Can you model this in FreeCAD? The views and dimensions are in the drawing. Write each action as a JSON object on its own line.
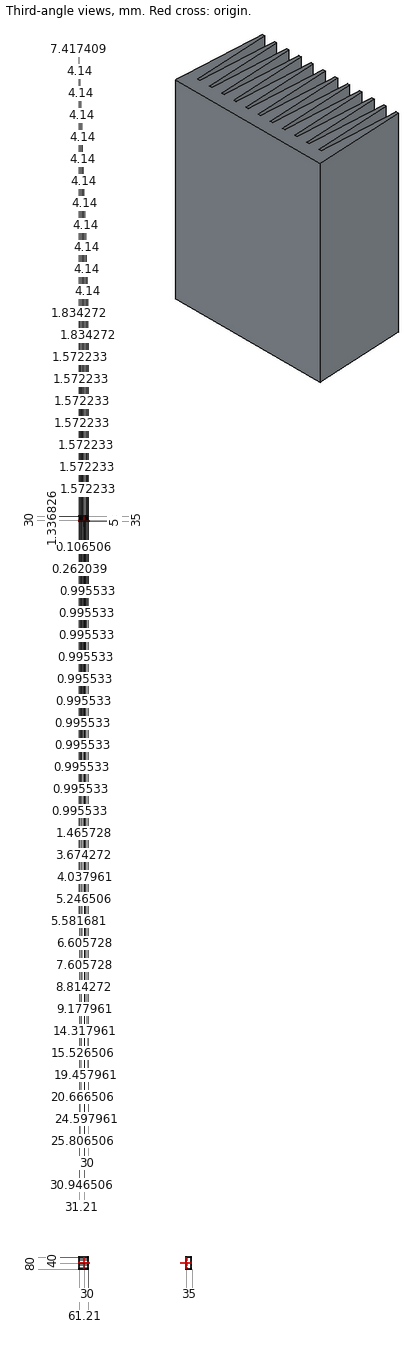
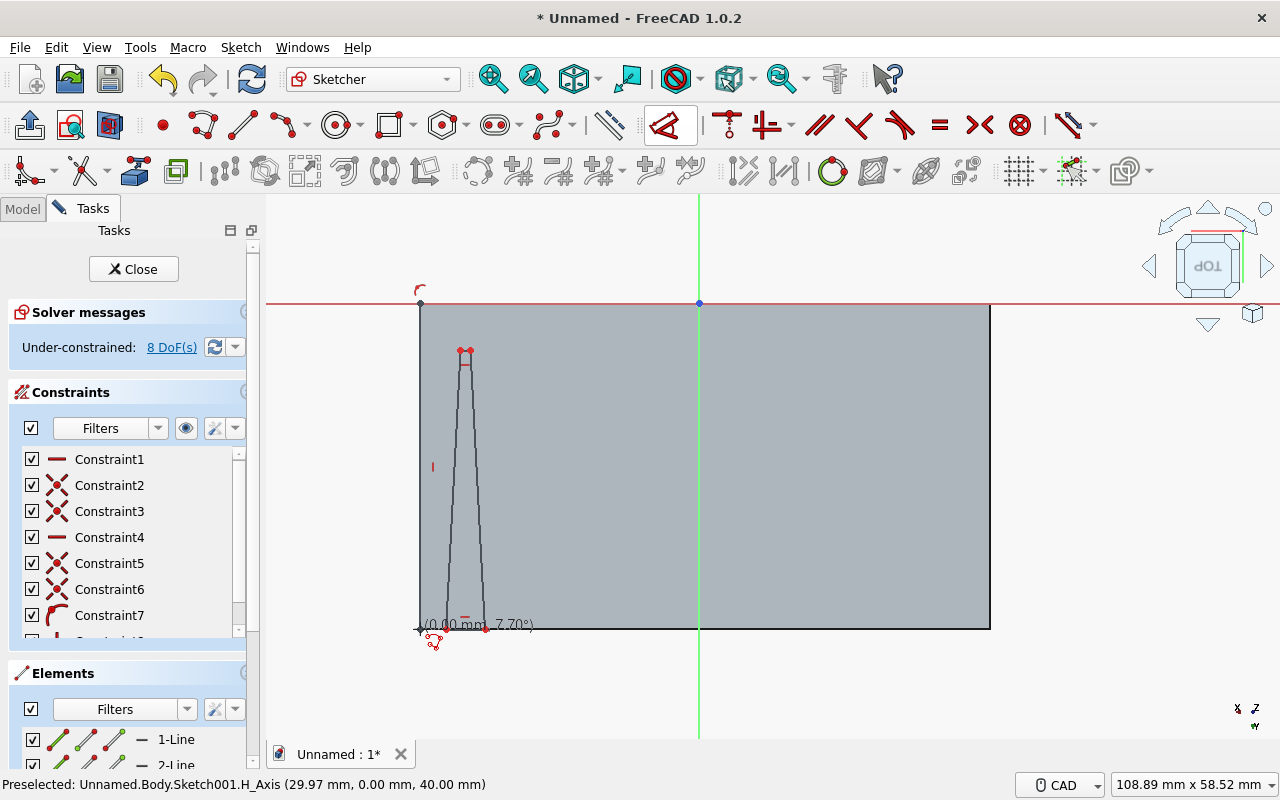
{"action": "scroll", "coordinate": [437, 629], "scroll_direction": "up", "scroll_amount": 3}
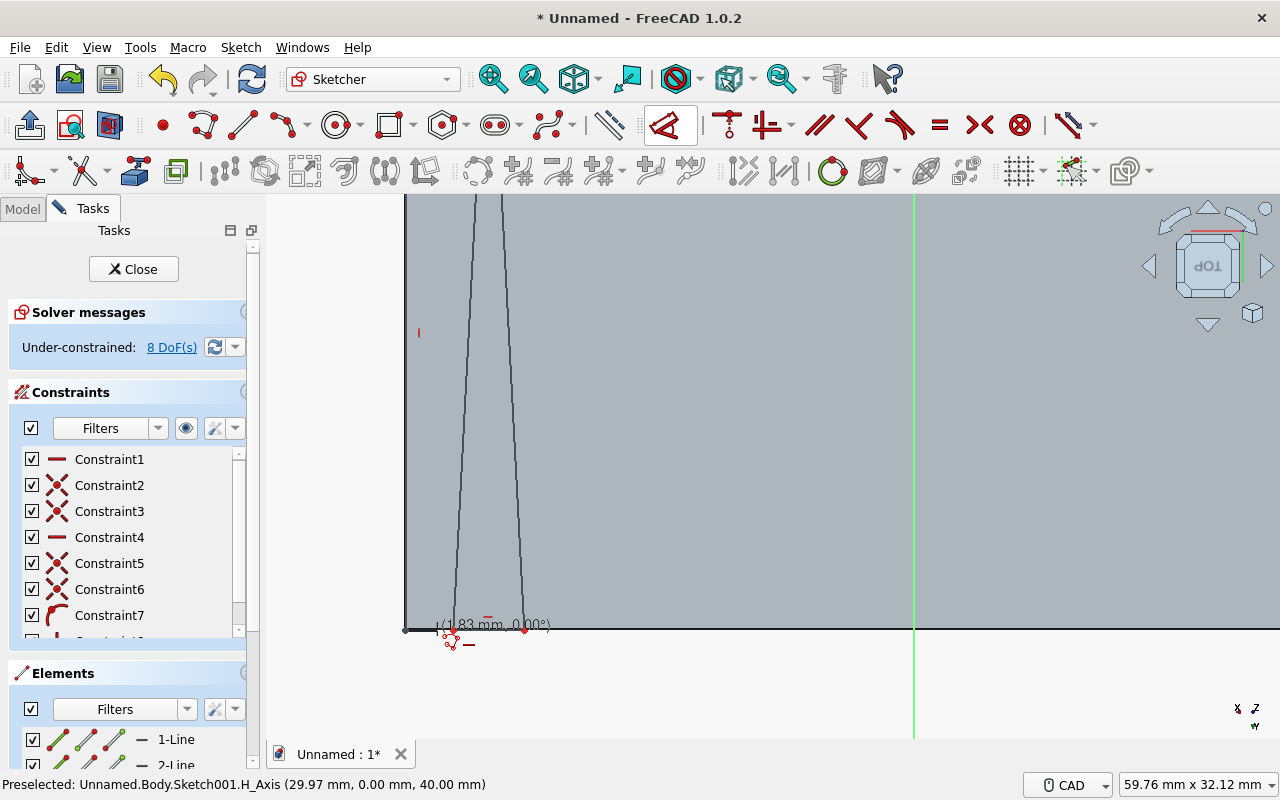
{"action": "left_click", "coordinate": [437, 628]}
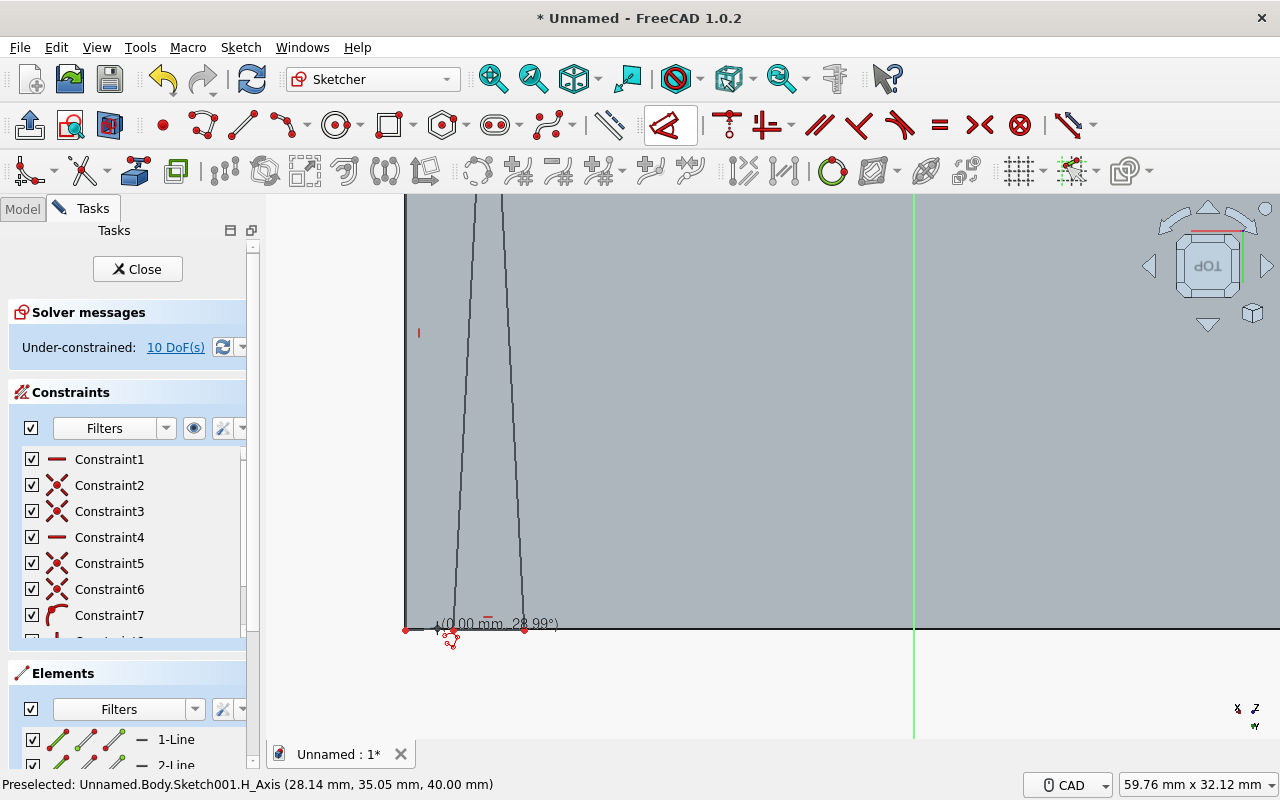
{"action": "scroll", "coordinate": [437, 630], "scroll_direction": "down", "scroll_amount": 3}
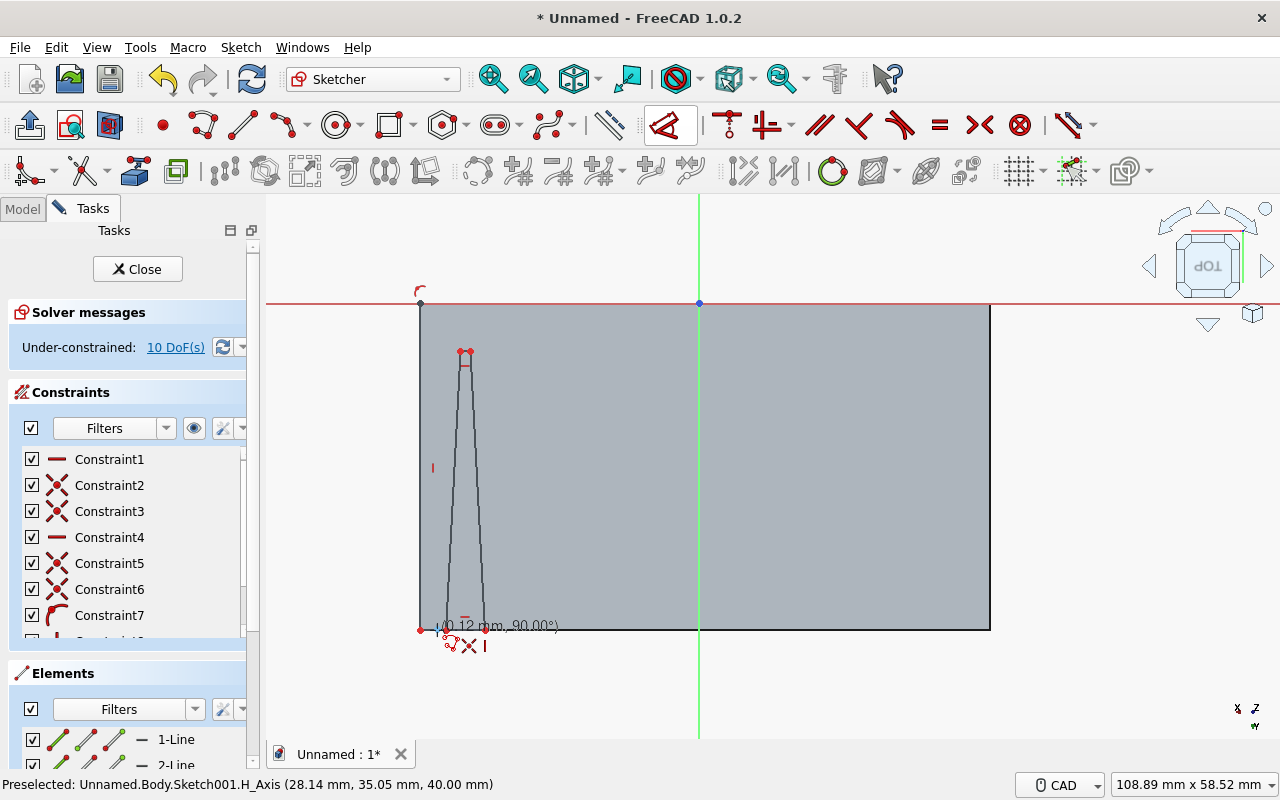
{"action": "left_click", "coordinate": [420, 304]}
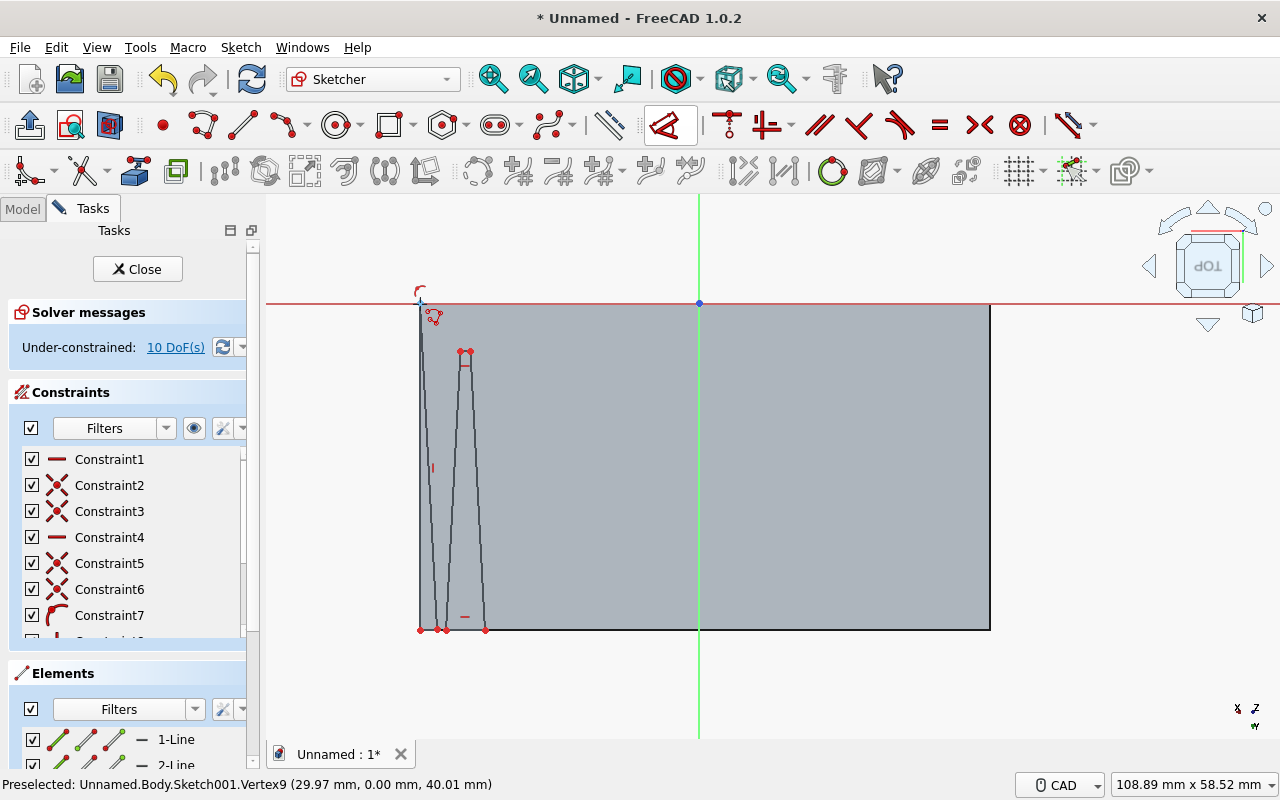
{"action": "left_click", "coordinate": [518, 351]}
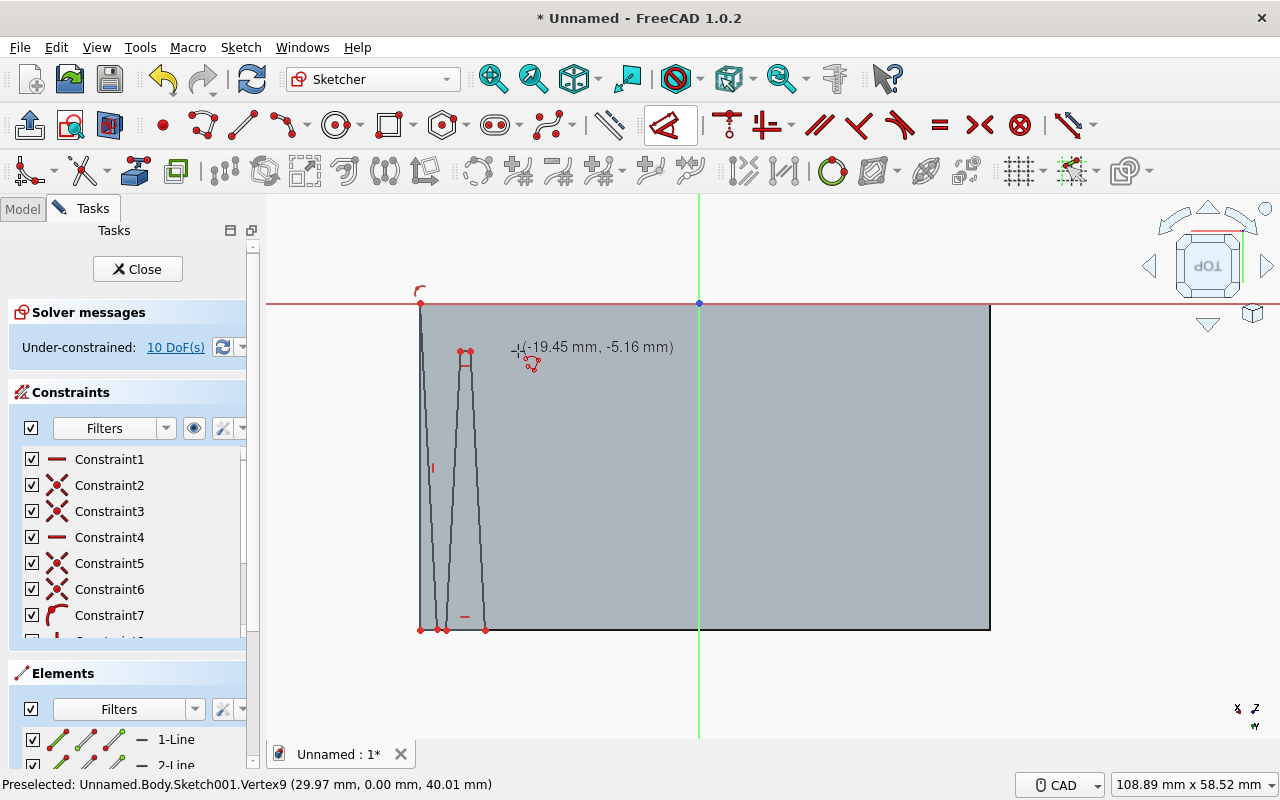
{"action": "scroll", "coordinate": [509, 351], "scroll_direction": "up", "scroll_amount": 3}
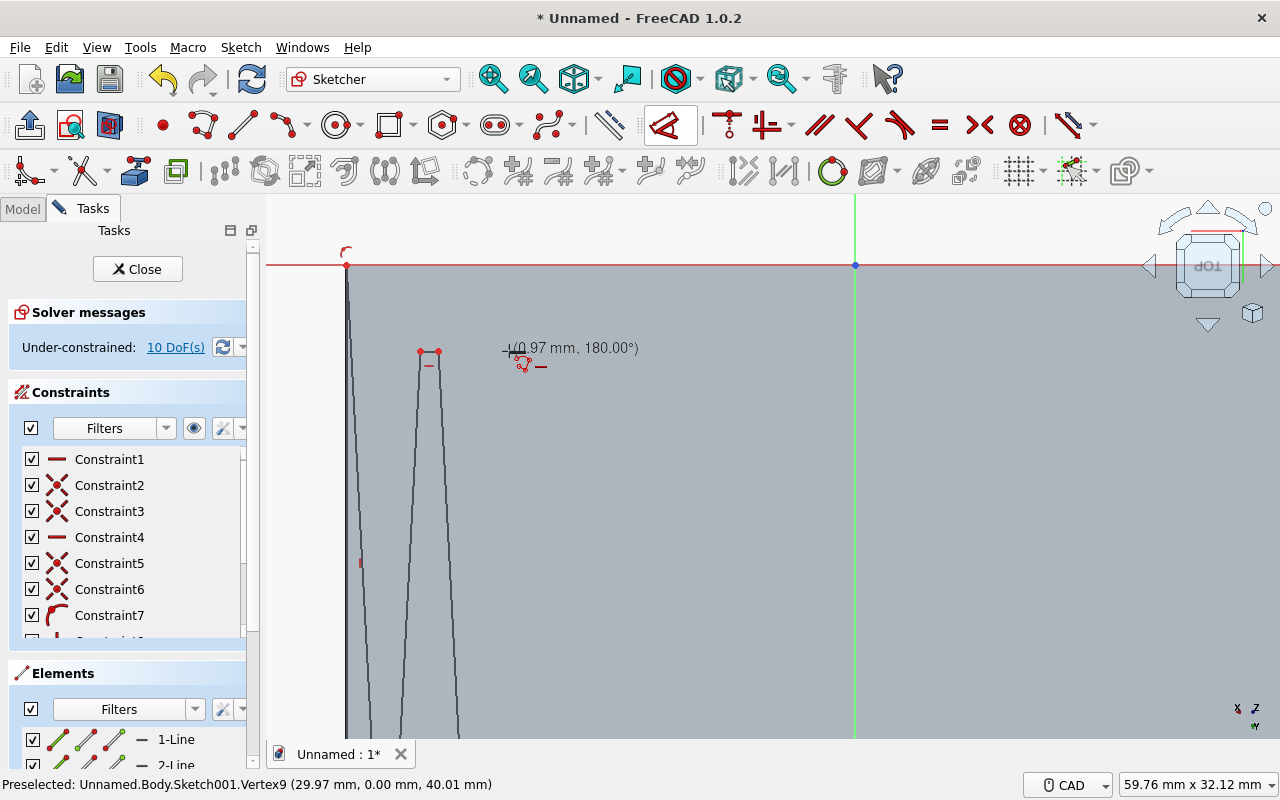
{"action": "left_click", "coordinate": [508, 351]}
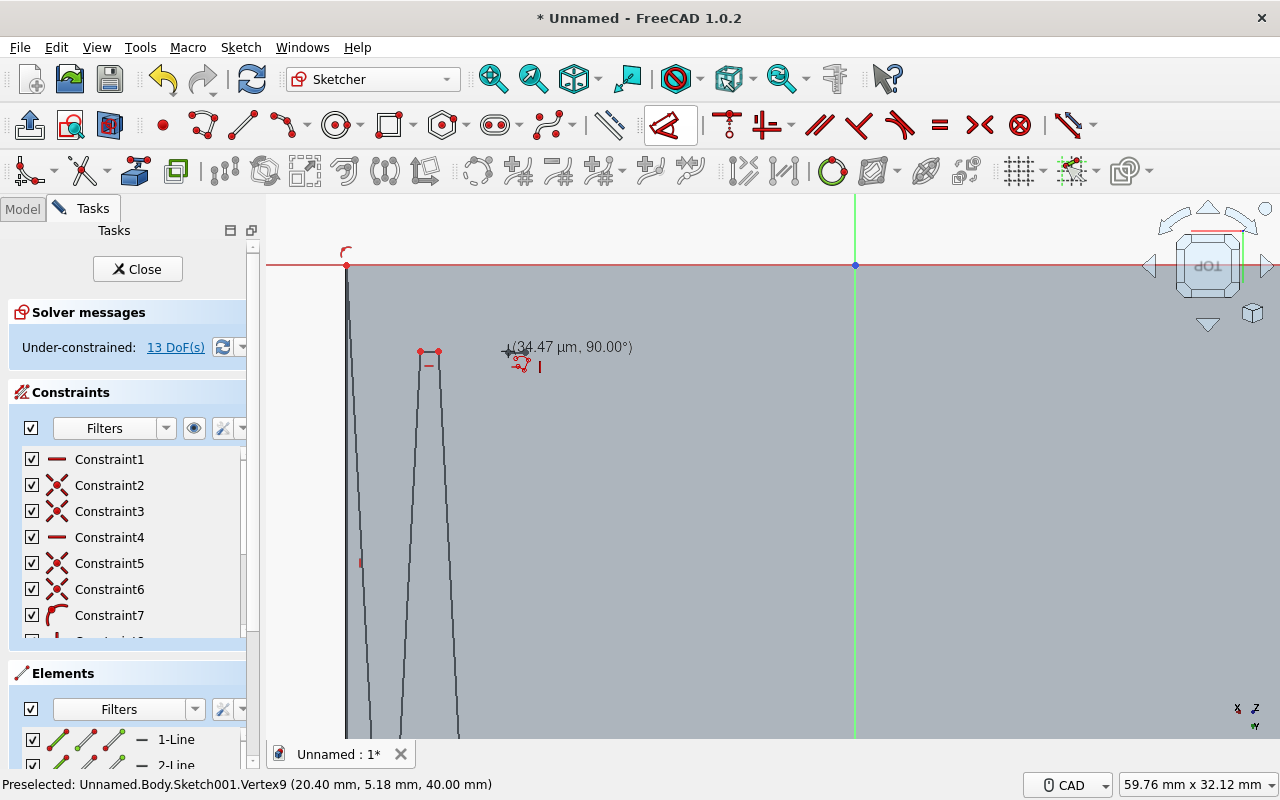
{"action": "scroll", "coordinate": [509, 350], "scroll_direction": "down", "scroll_amount": 3}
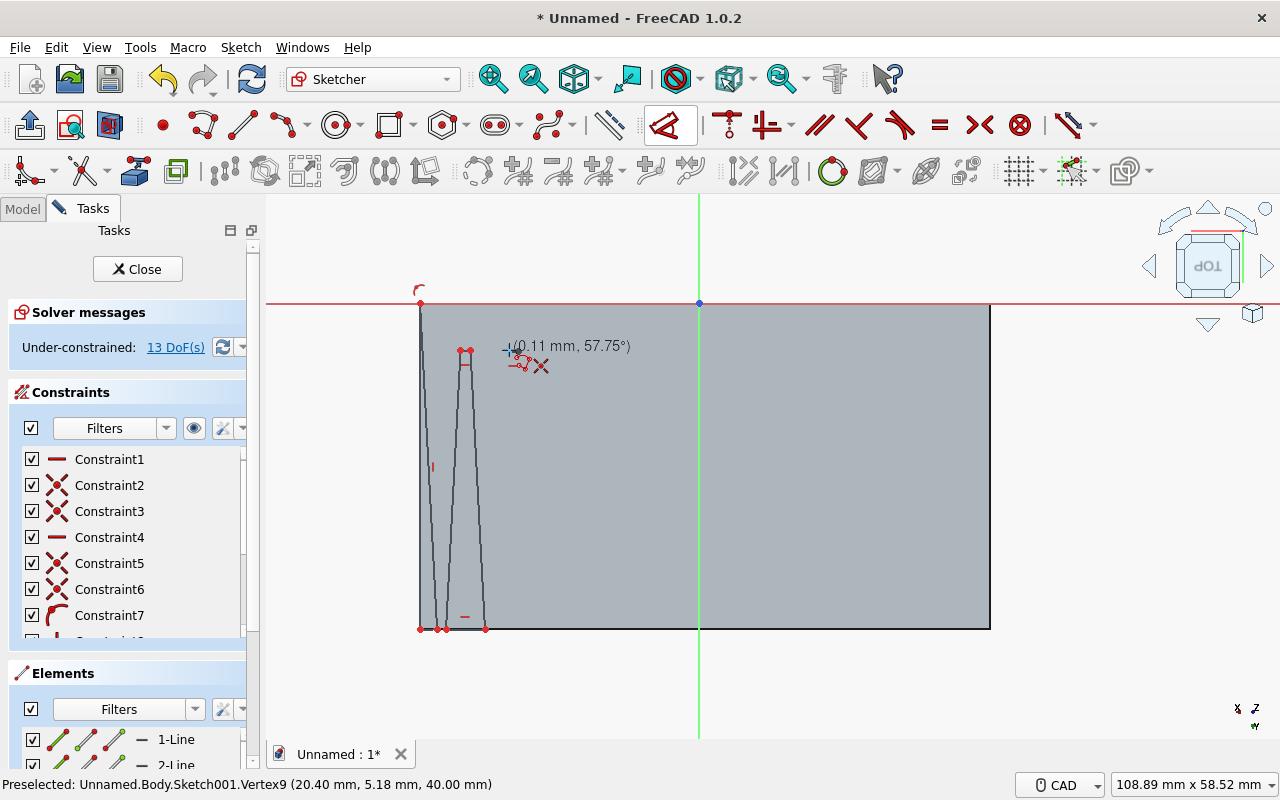
{"action": "scroll", "coordinate": [494, 629], "scroll_direction": "up", "scroll_amount": 3}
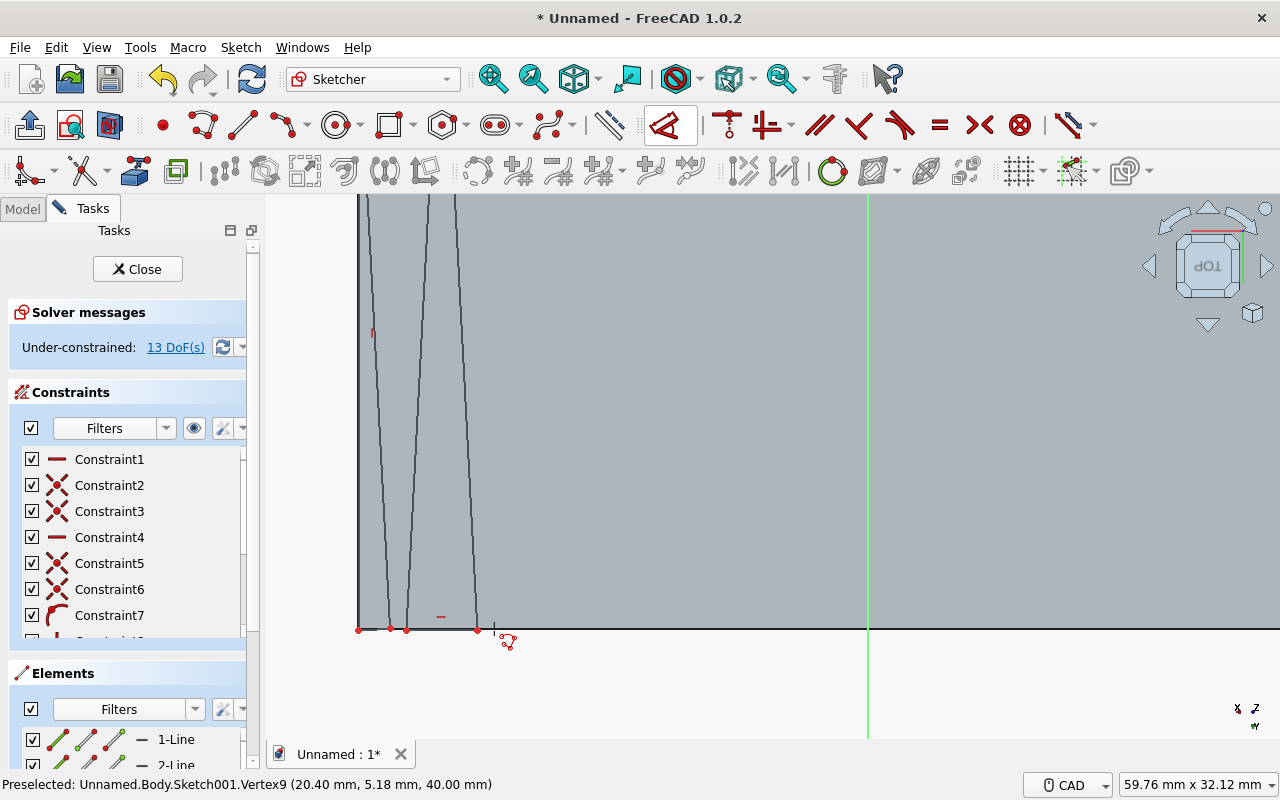
{"action": "left_click", "coordinate": [494, 629]}
{"action": "left_click", "coordinate": [564, 629]}